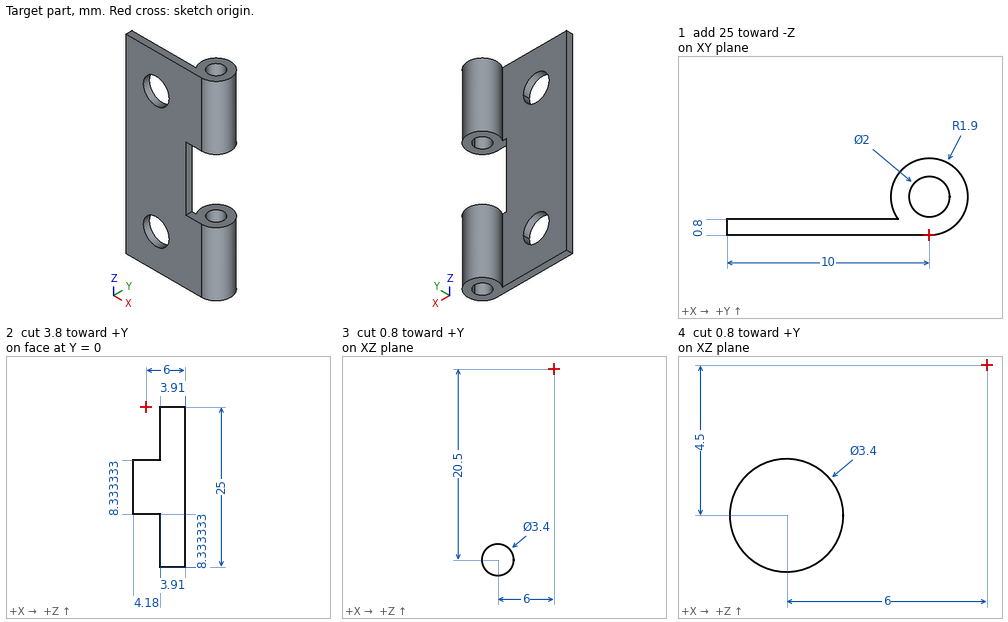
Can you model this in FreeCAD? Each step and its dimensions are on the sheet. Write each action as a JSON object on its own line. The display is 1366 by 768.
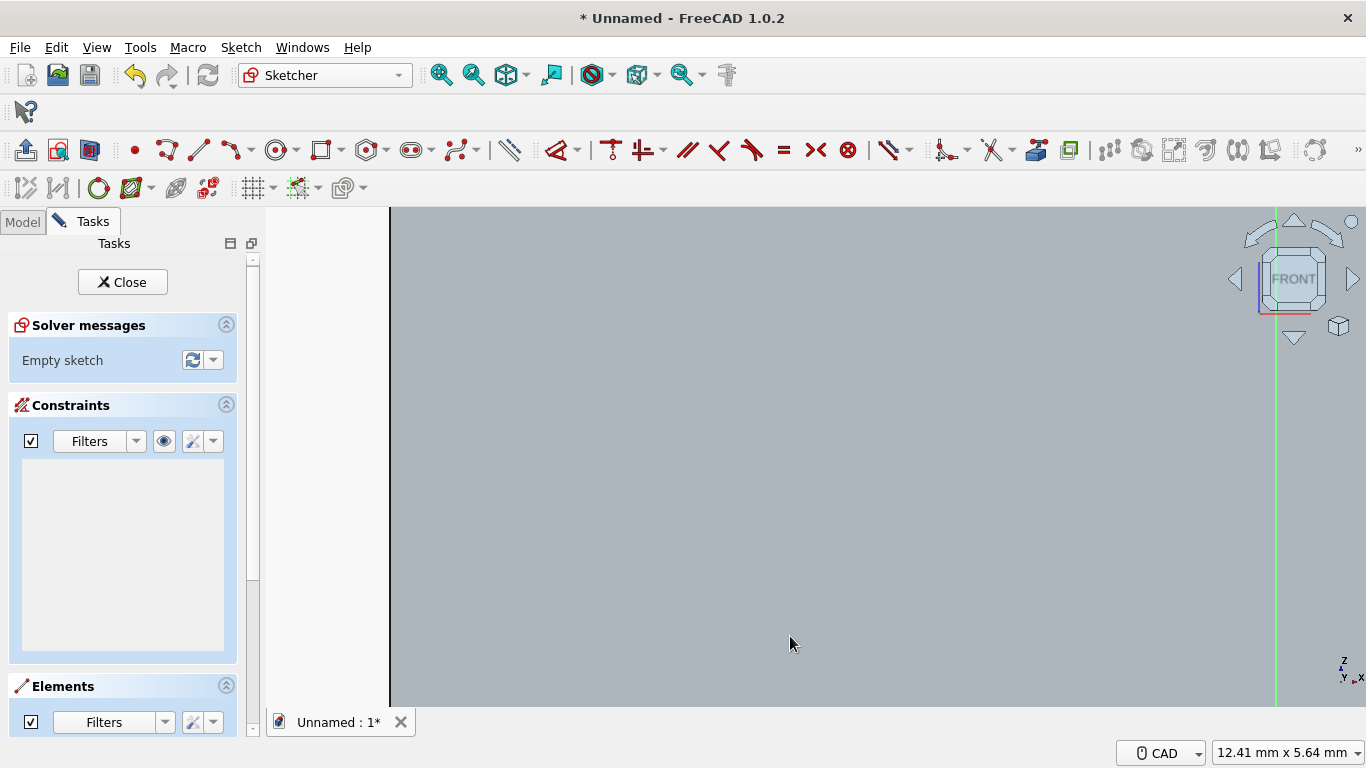
{"action": "left_click", "coordinate": [276, 150]}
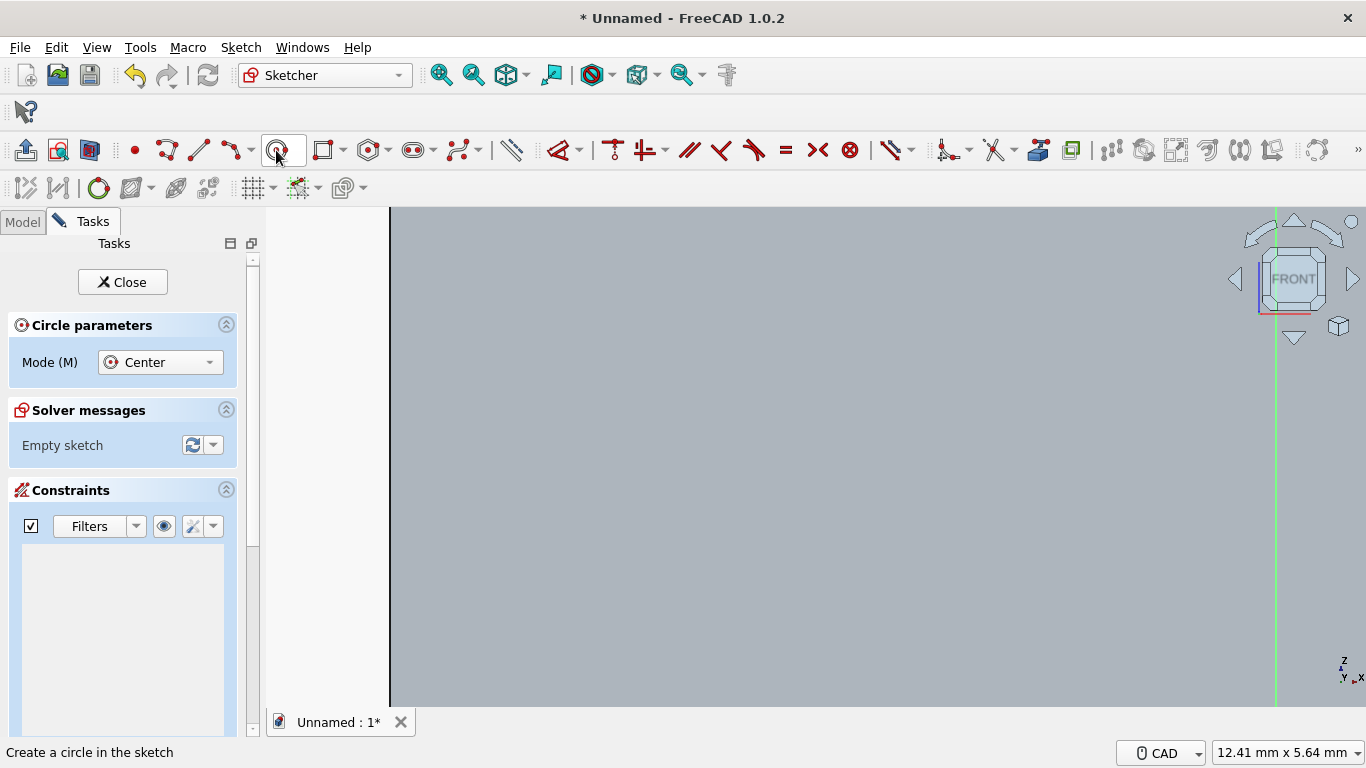
{"action": "left_click", "coordinate": [744, 455]}
{"action": "left_click", "coordinate": [851, 348]}
{"action": "key", "text": "Escape"}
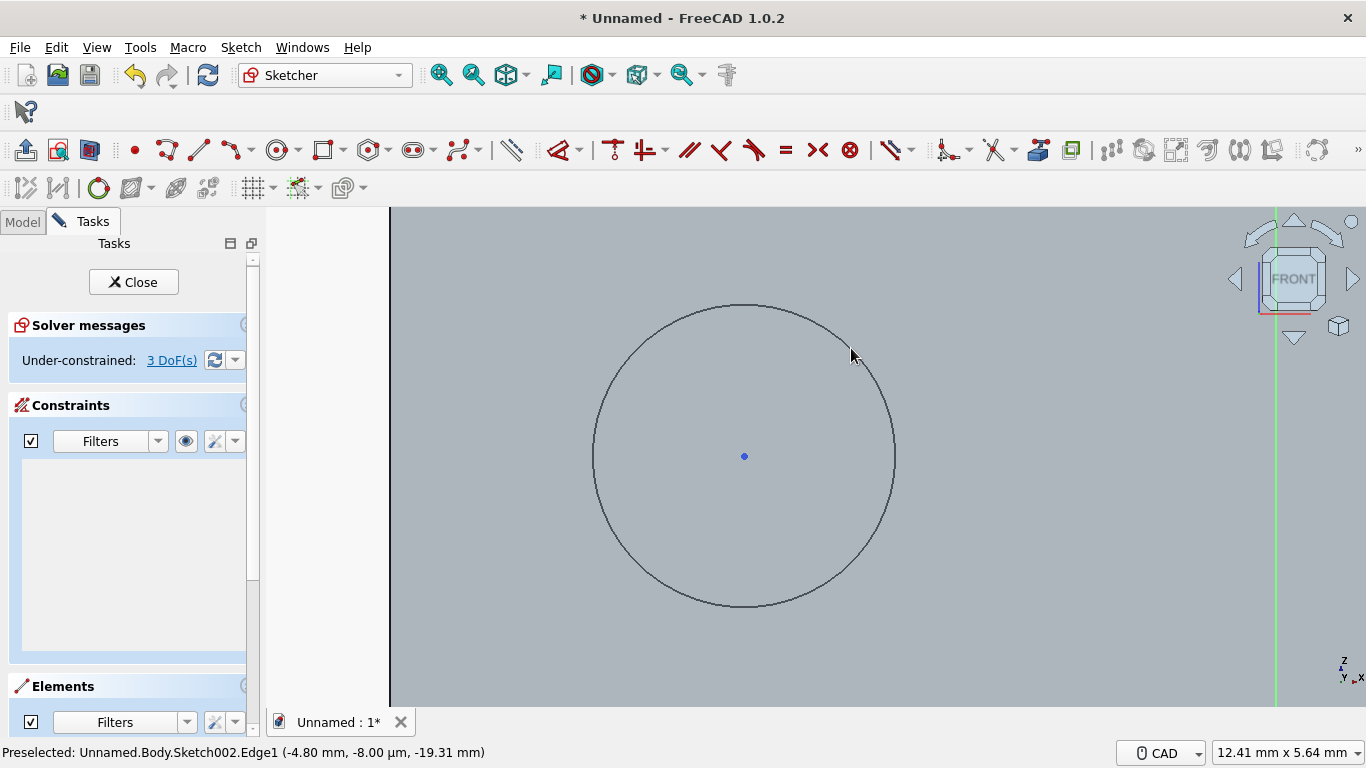
{"action": "left_click", "coordinate": [558, 150]}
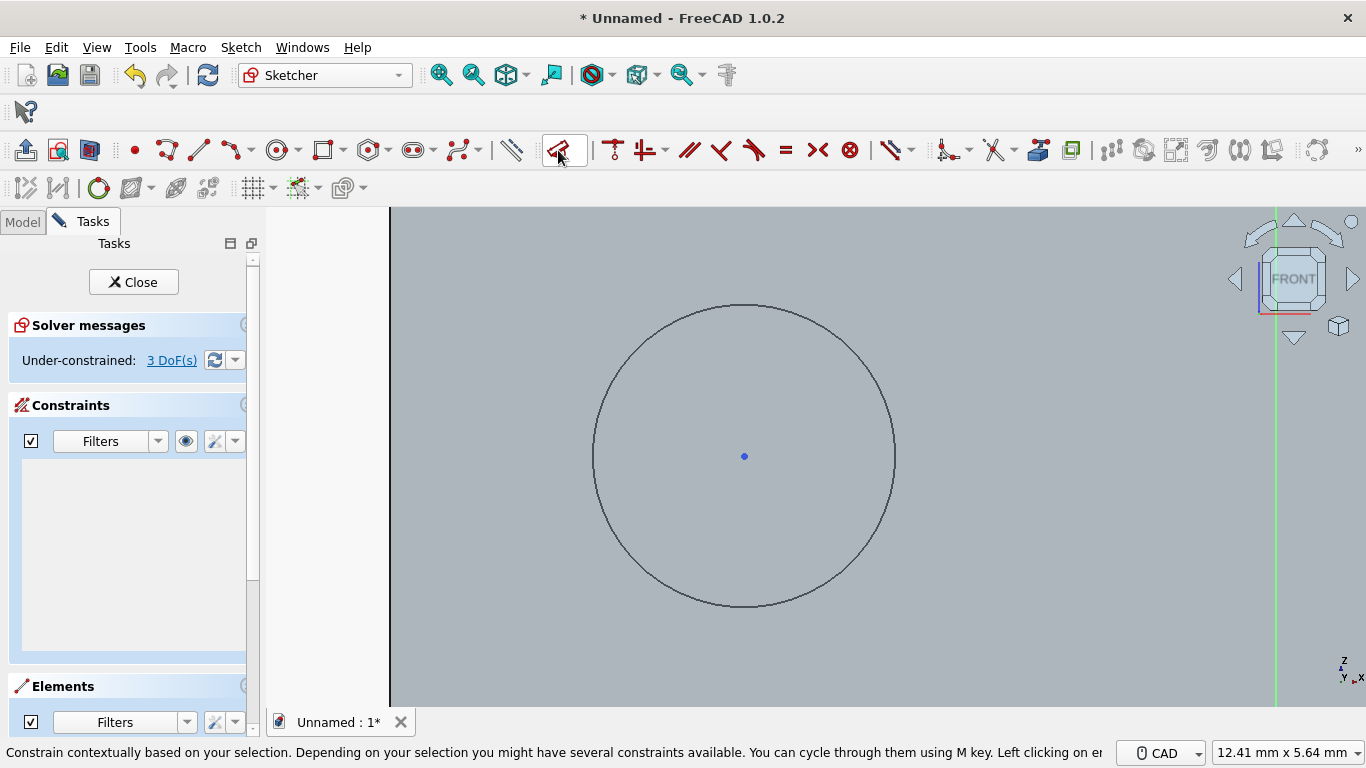
{"action": "left_click", "coordinate": [851, 349]}
{"action": "left_click", "coordinate": [874, 326]}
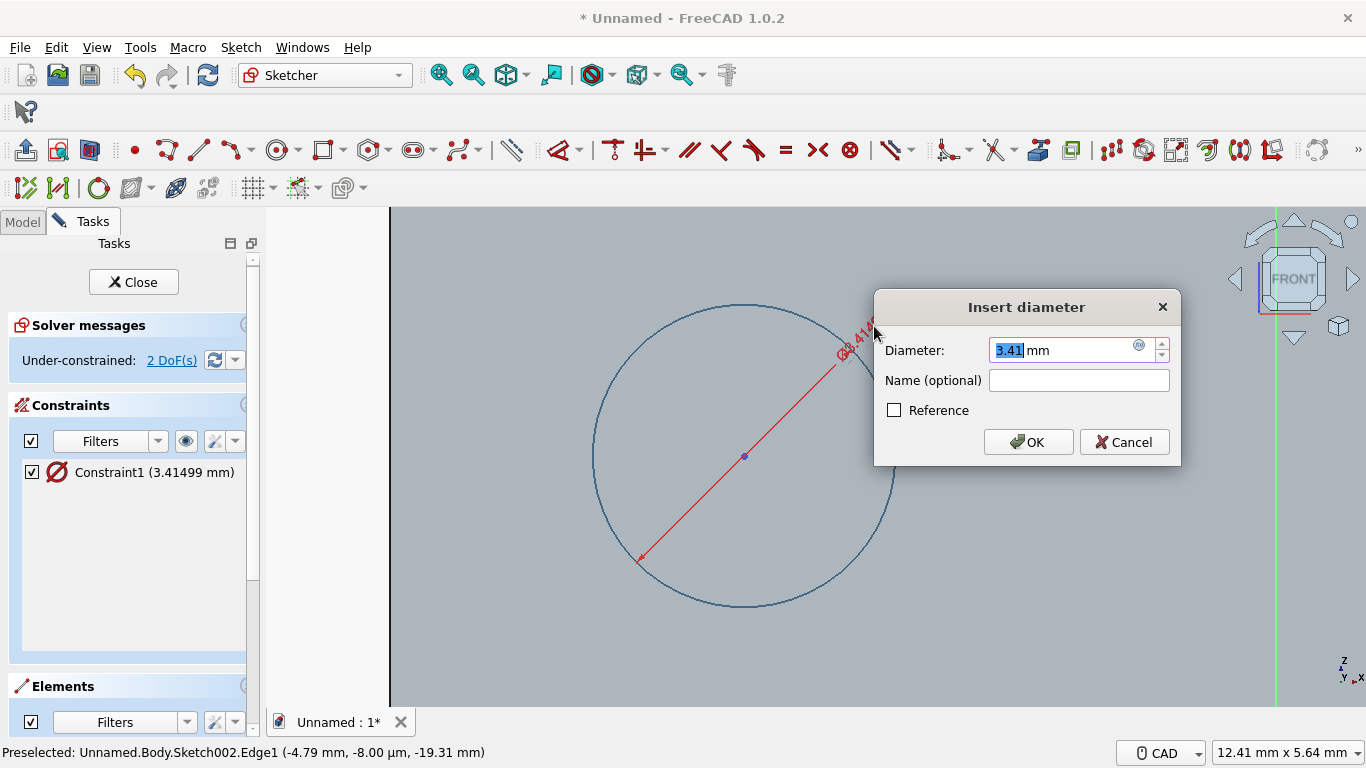
{"action": "type", "text": "3.4"}
{"action": "key", "text": "Return"}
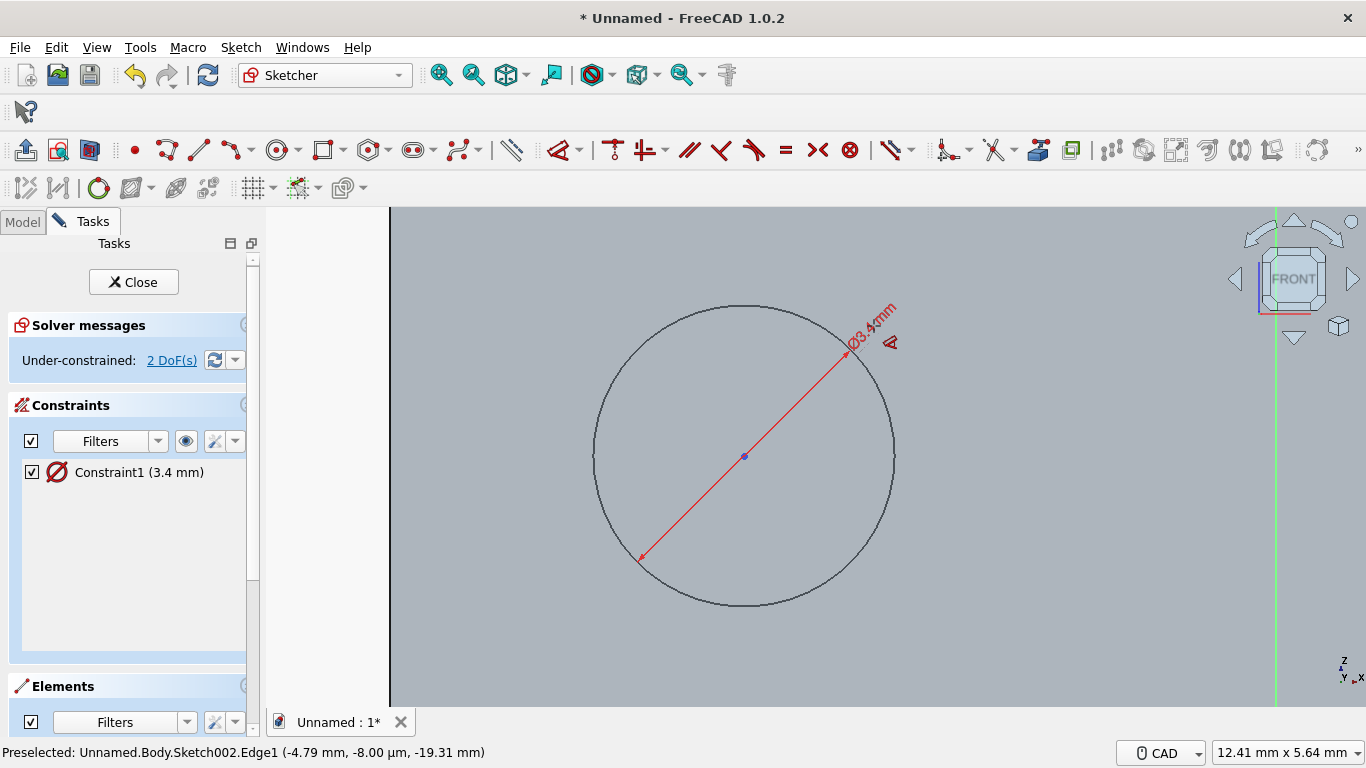
{"action": "left_click", "coordinate": [744, 456]}
{"action": "left_click", "coordinate": [973, 490]}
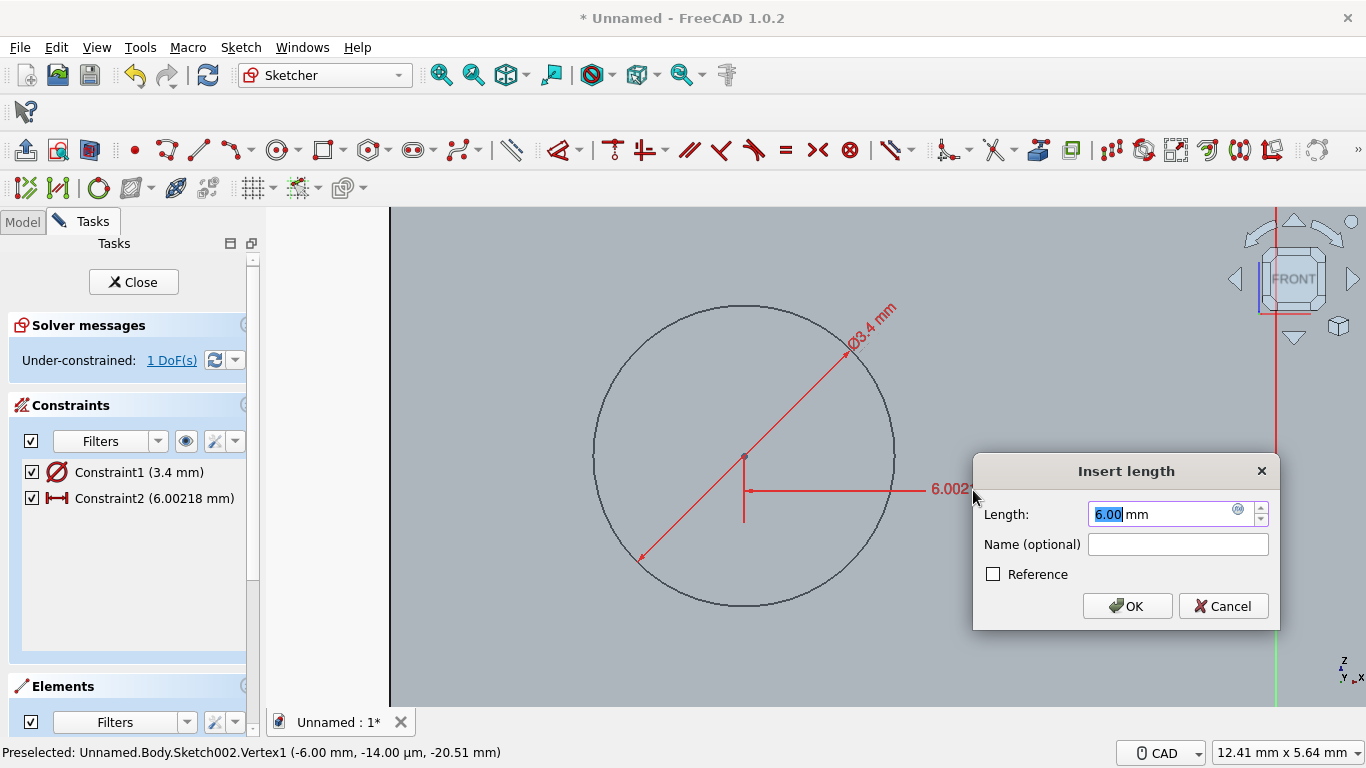
{"action": "type", "text": "6"}
{"action": "key", "text": "Return"}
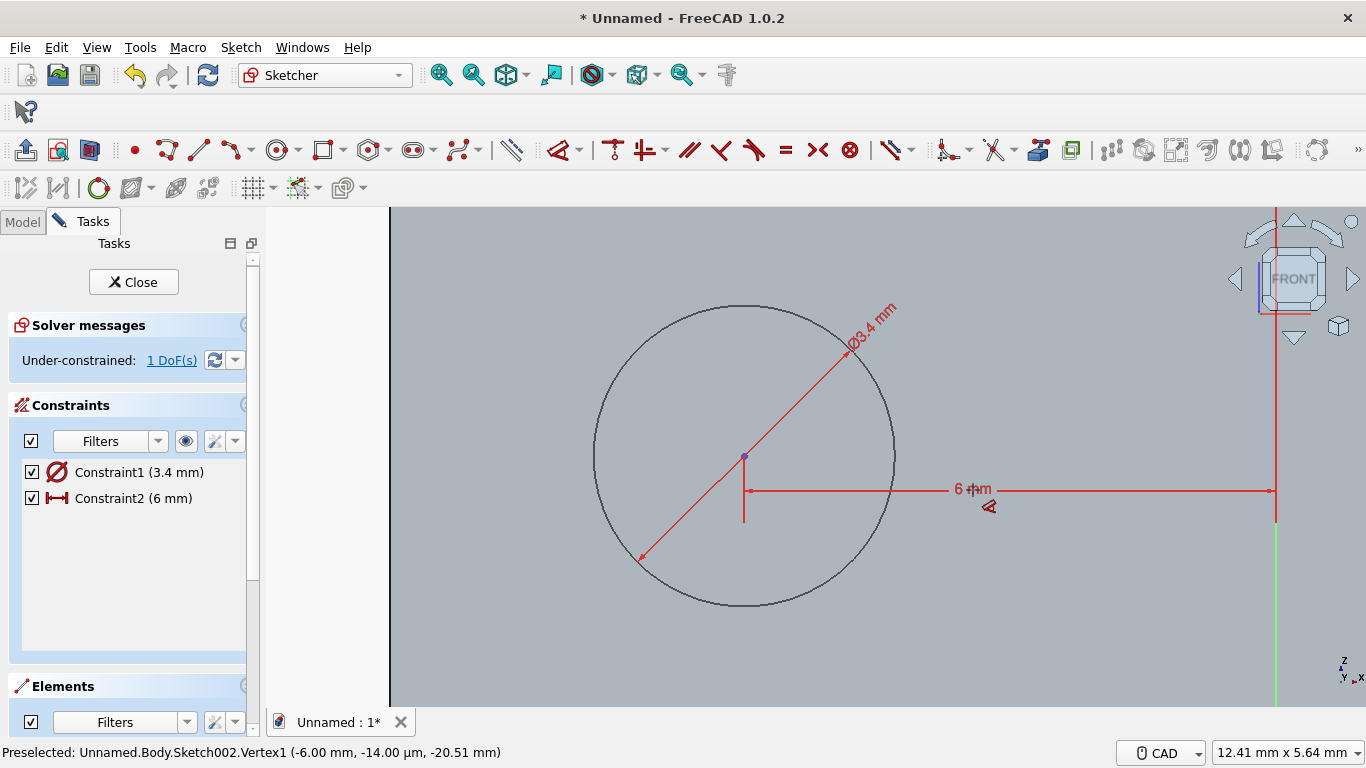
{"action": "left_click", "coordinate": [744, 456]}
{"action": "left_click", "coordinate": [710, 346]}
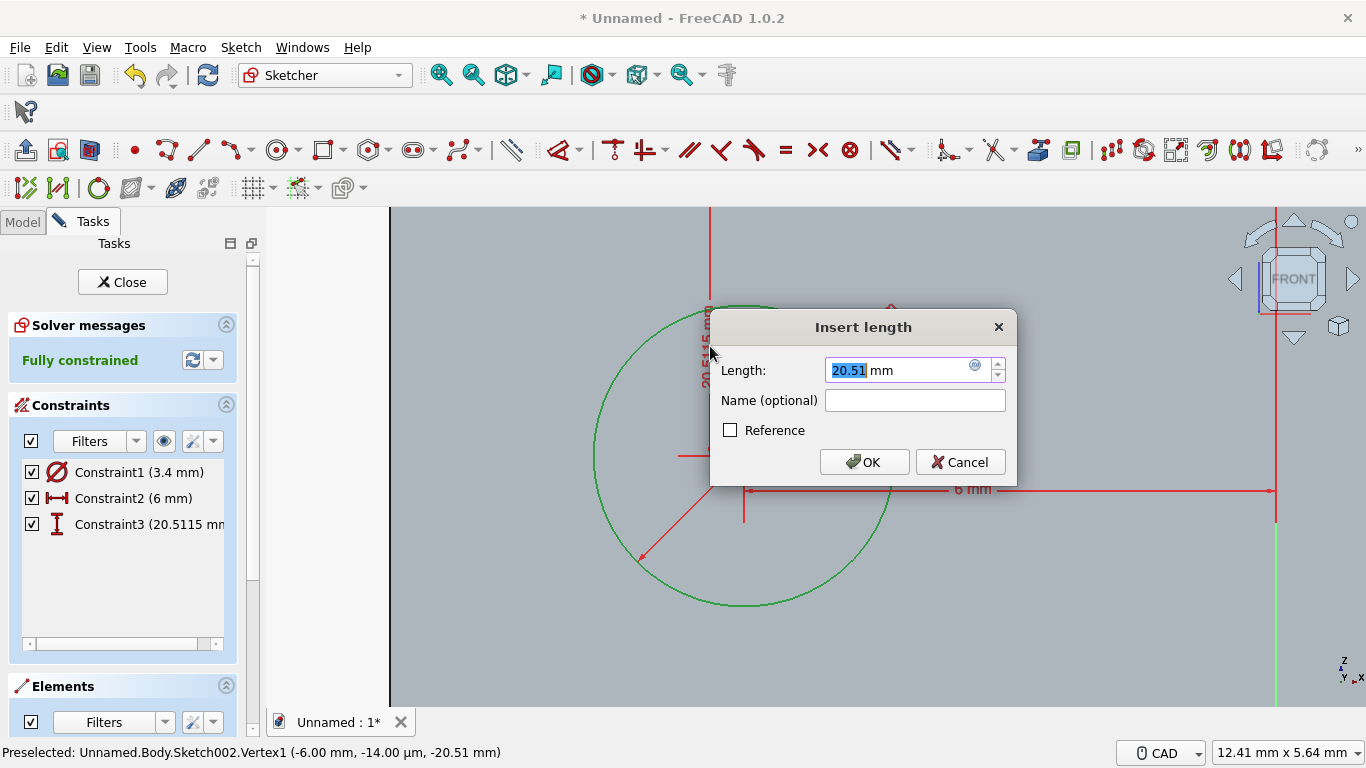
{"action": "type", "text": "20.5"}
{"action": "key", "text": "Return"}
{"action": "key", "text": "Escape"}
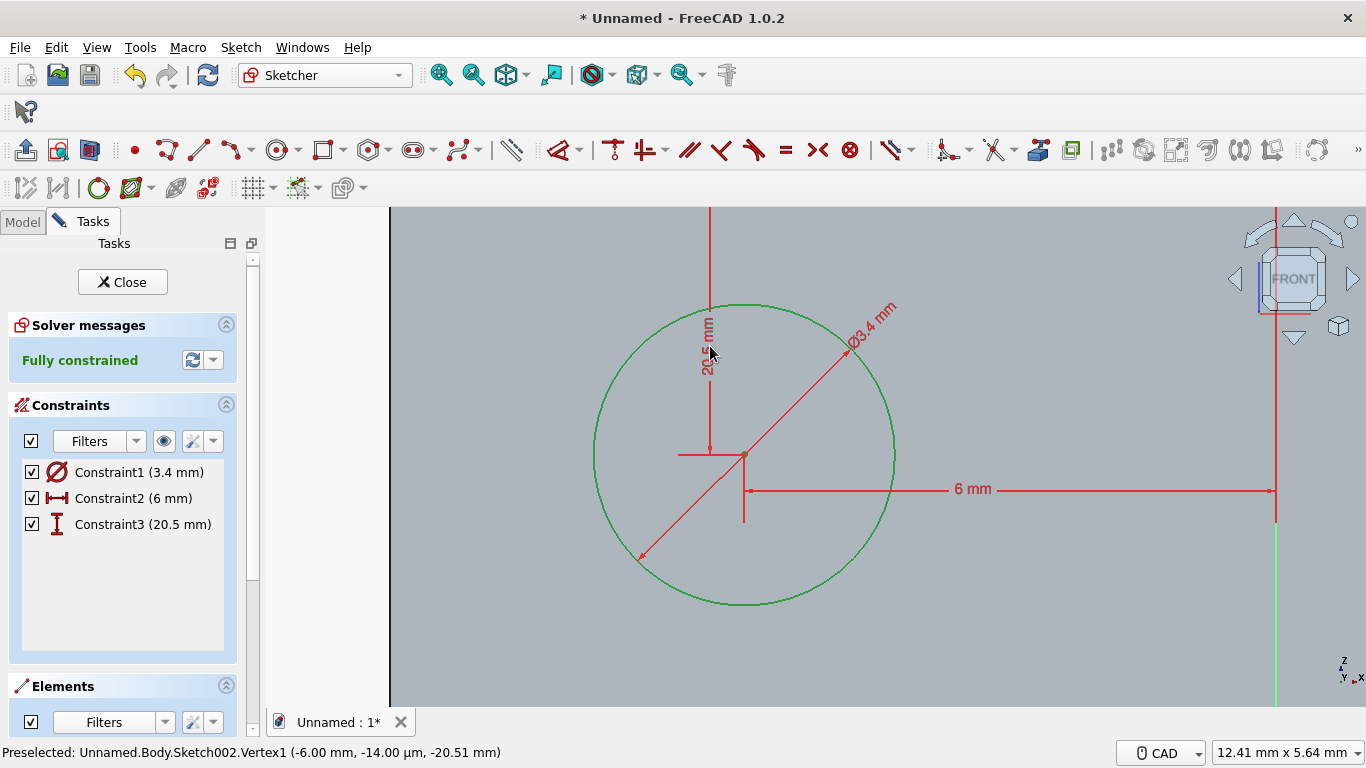
{"action": "left_click", "coordinate": [123, 282]}